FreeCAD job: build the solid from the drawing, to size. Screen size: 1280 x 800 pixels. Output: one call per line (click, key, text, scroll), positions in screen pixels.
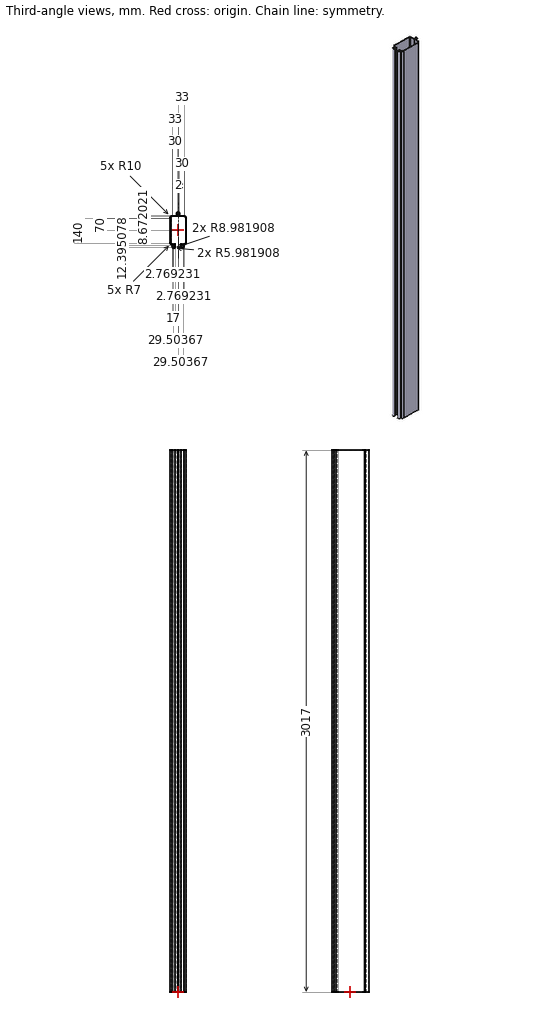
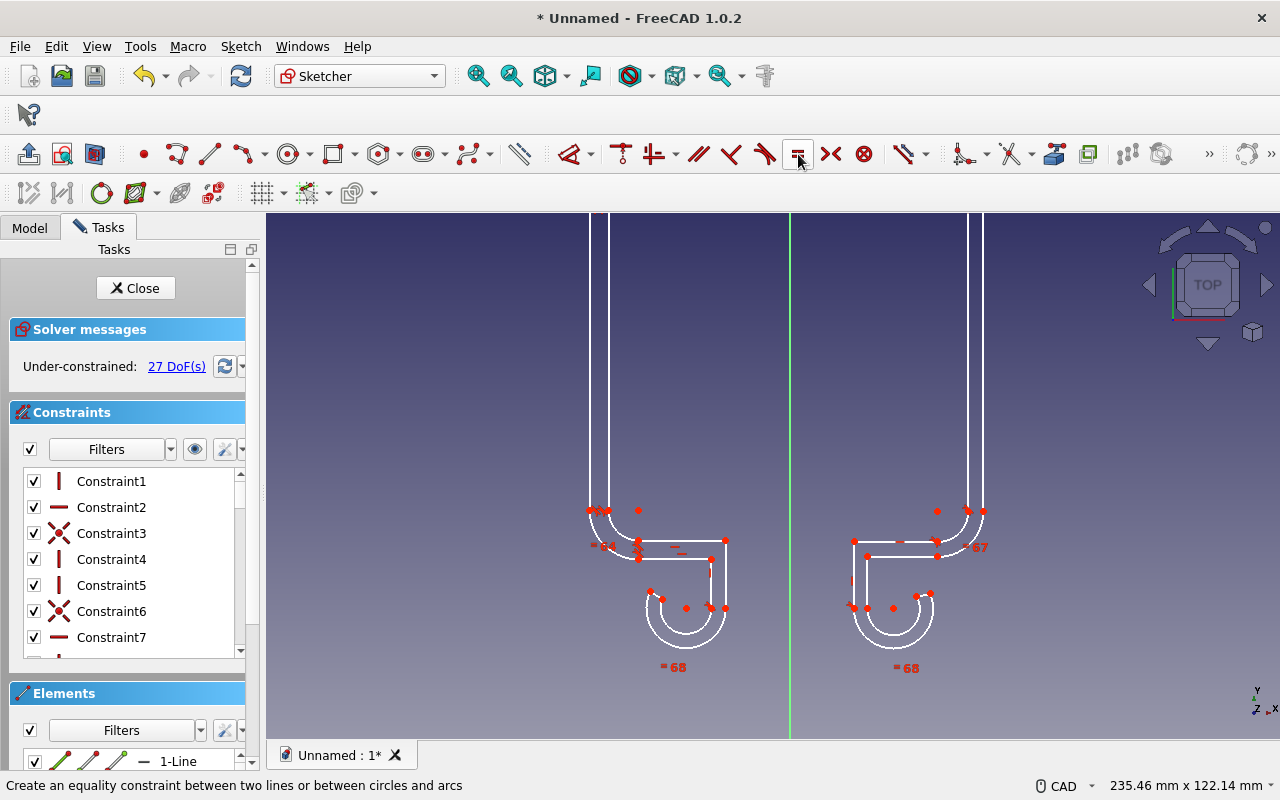
click(666, 625)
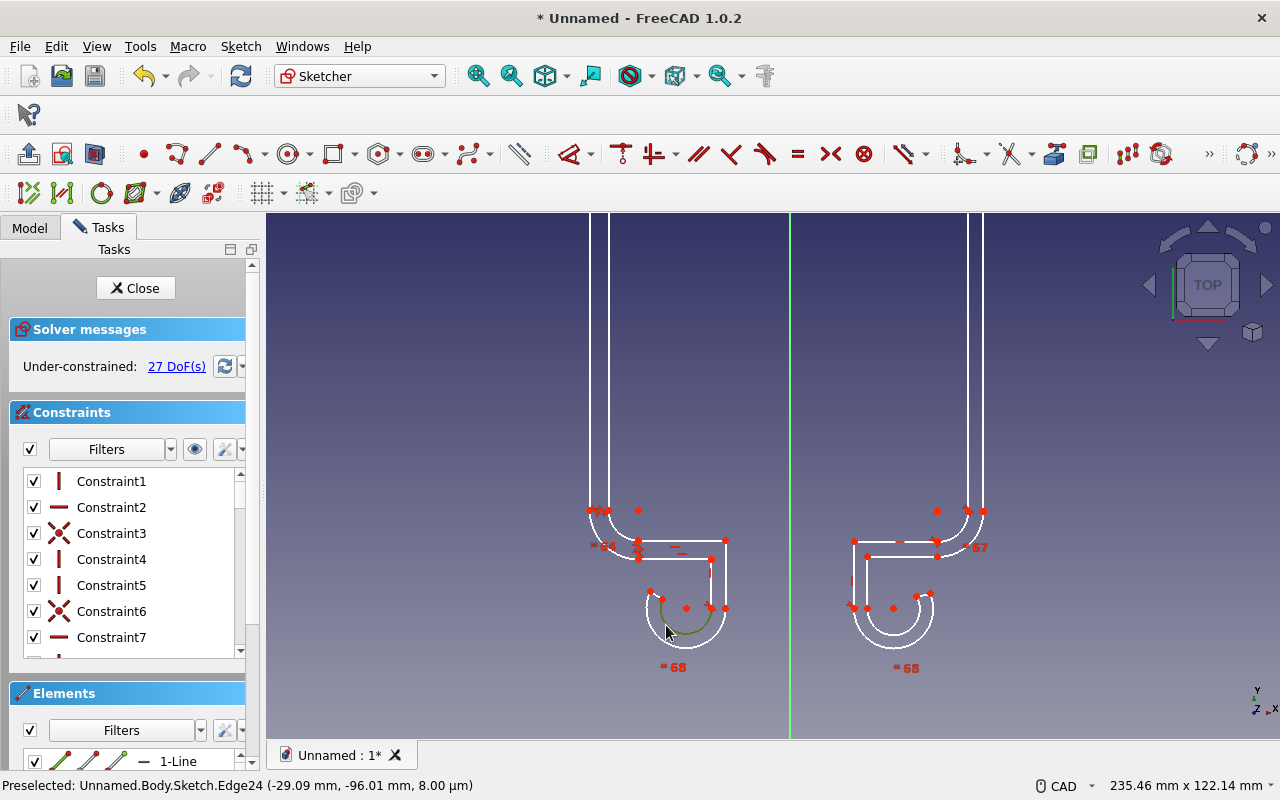
click(881, 632)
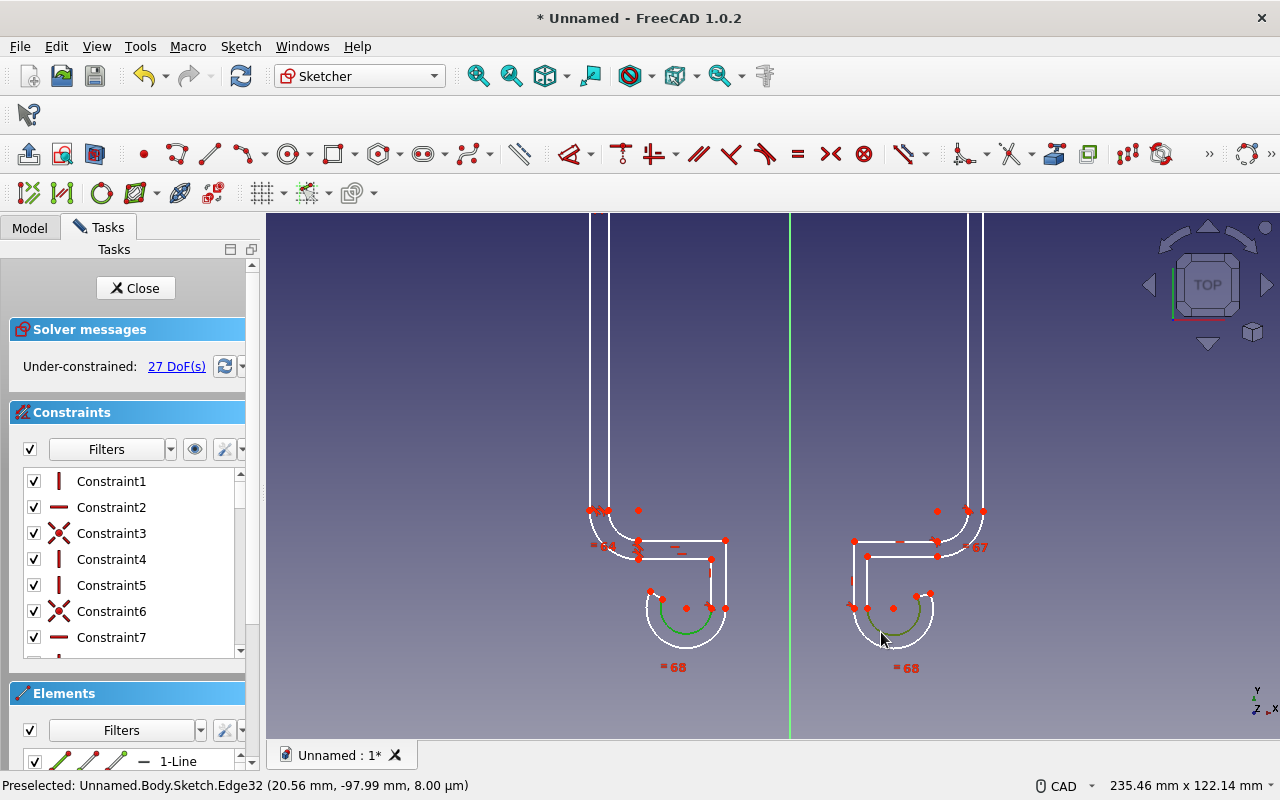
click(798, 154)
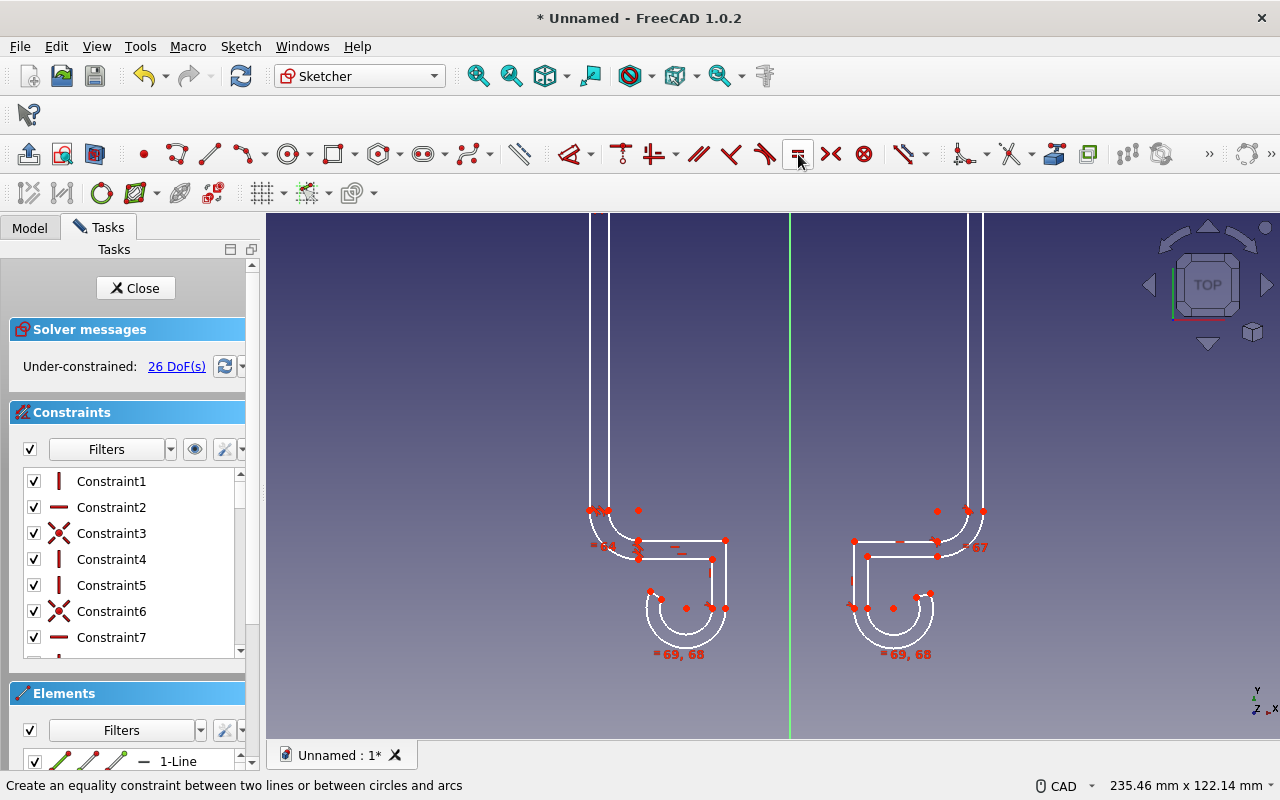
click(595, 533)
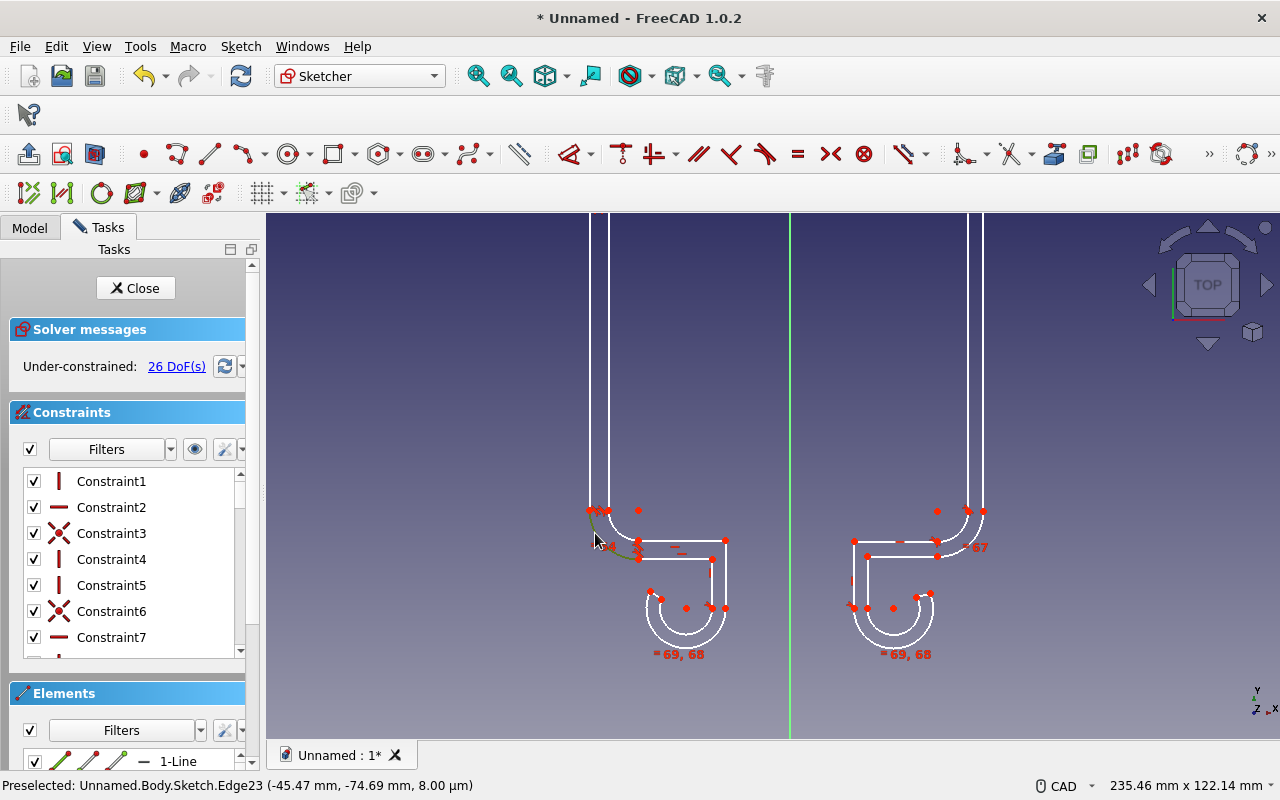
click(959, 552)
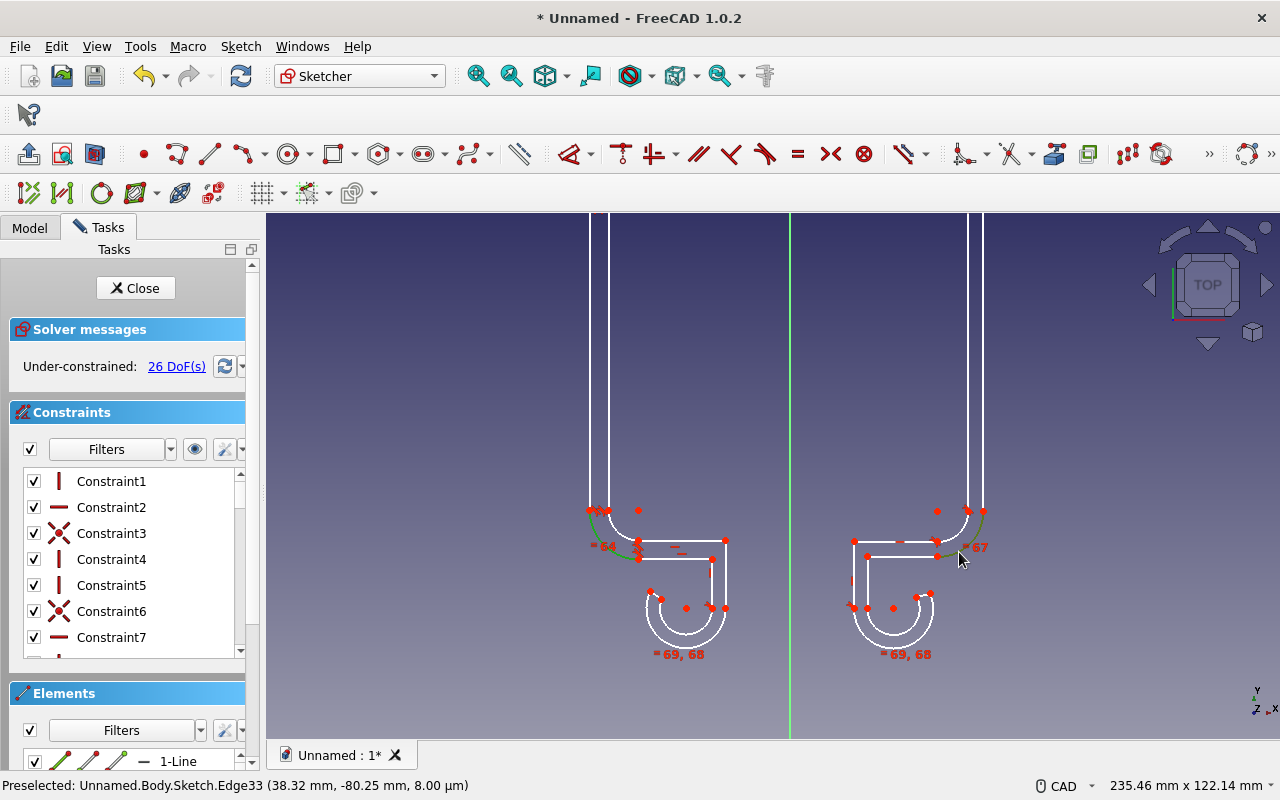
scroll(655, 633, down, 5)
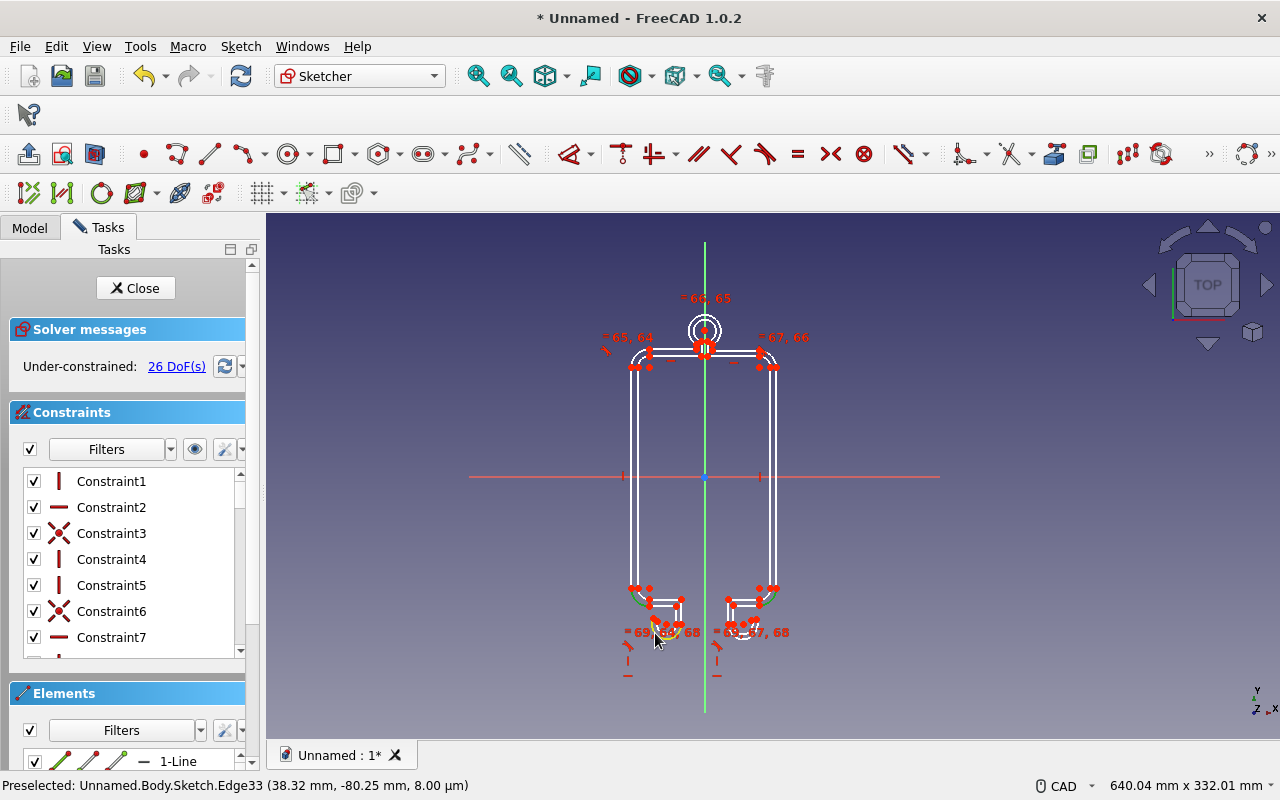
scroll(719, 323, up, 6)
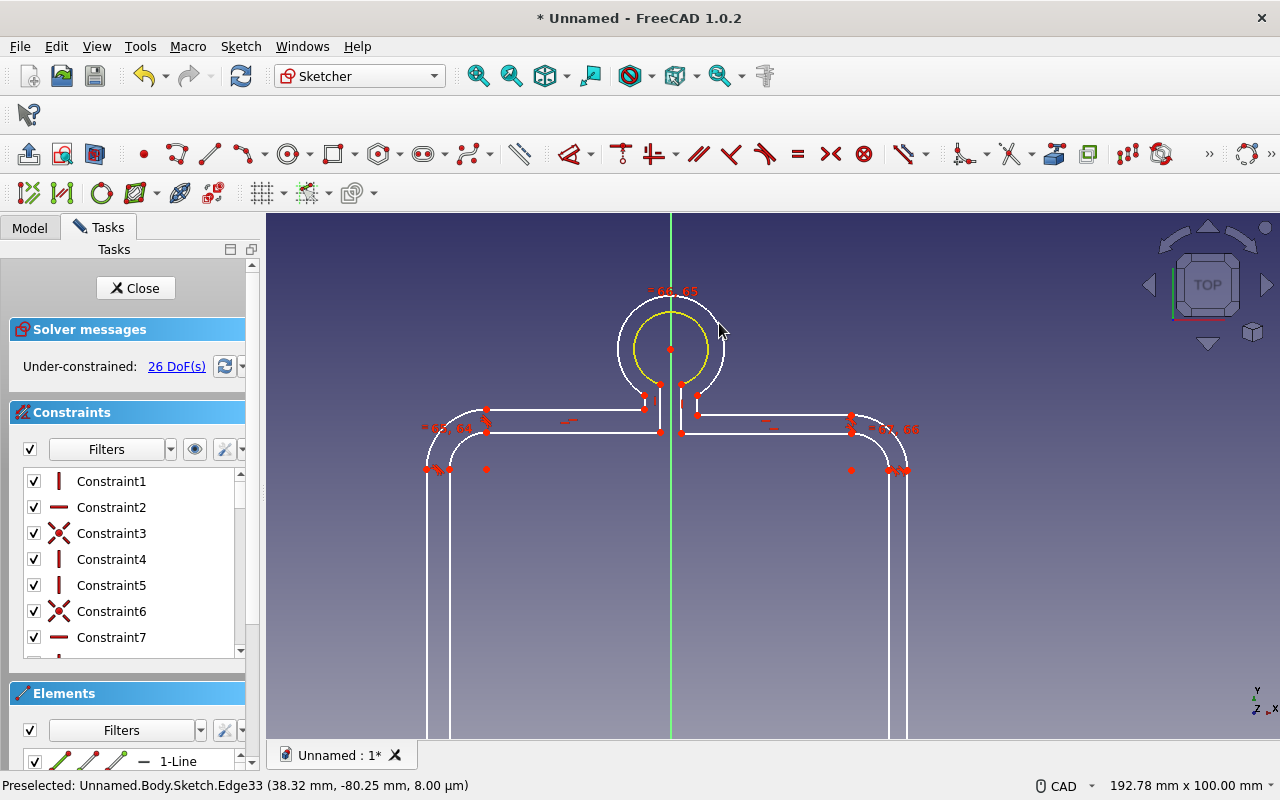
click(717, 323)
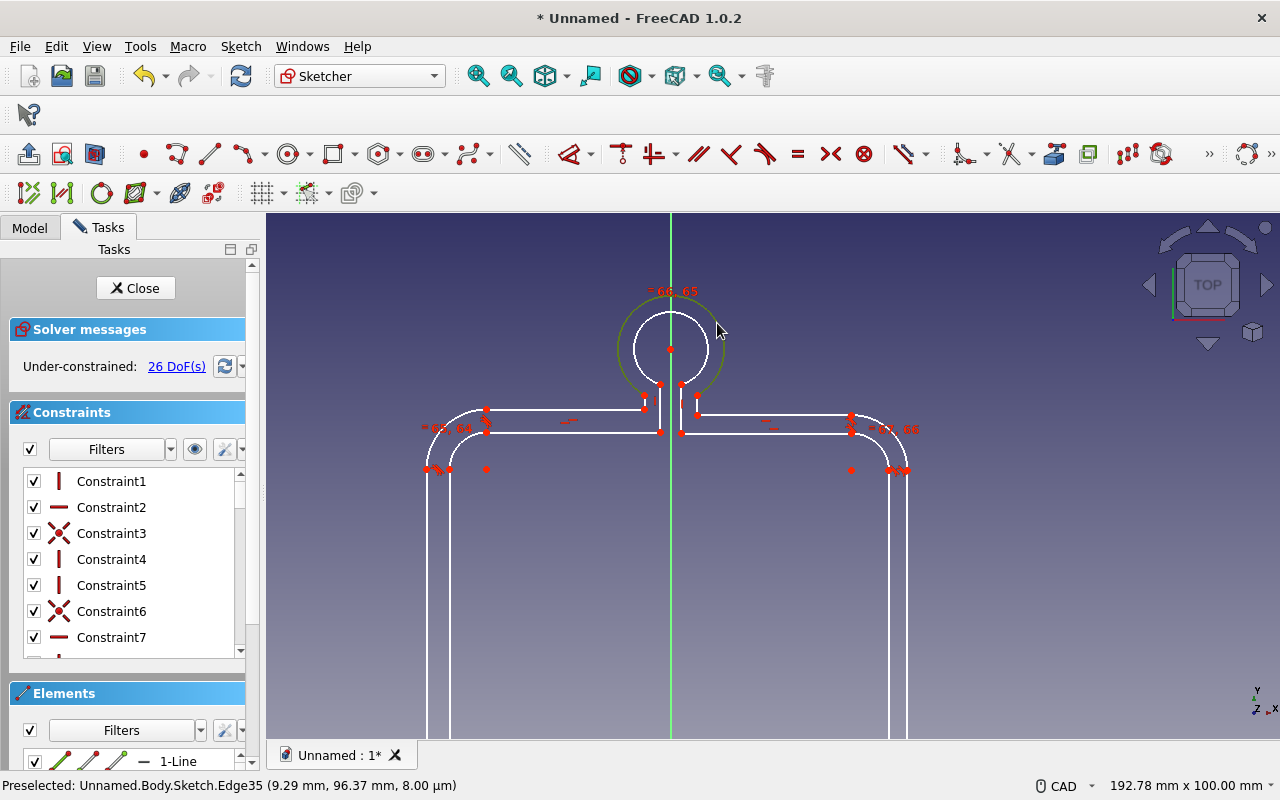
click(798, 154)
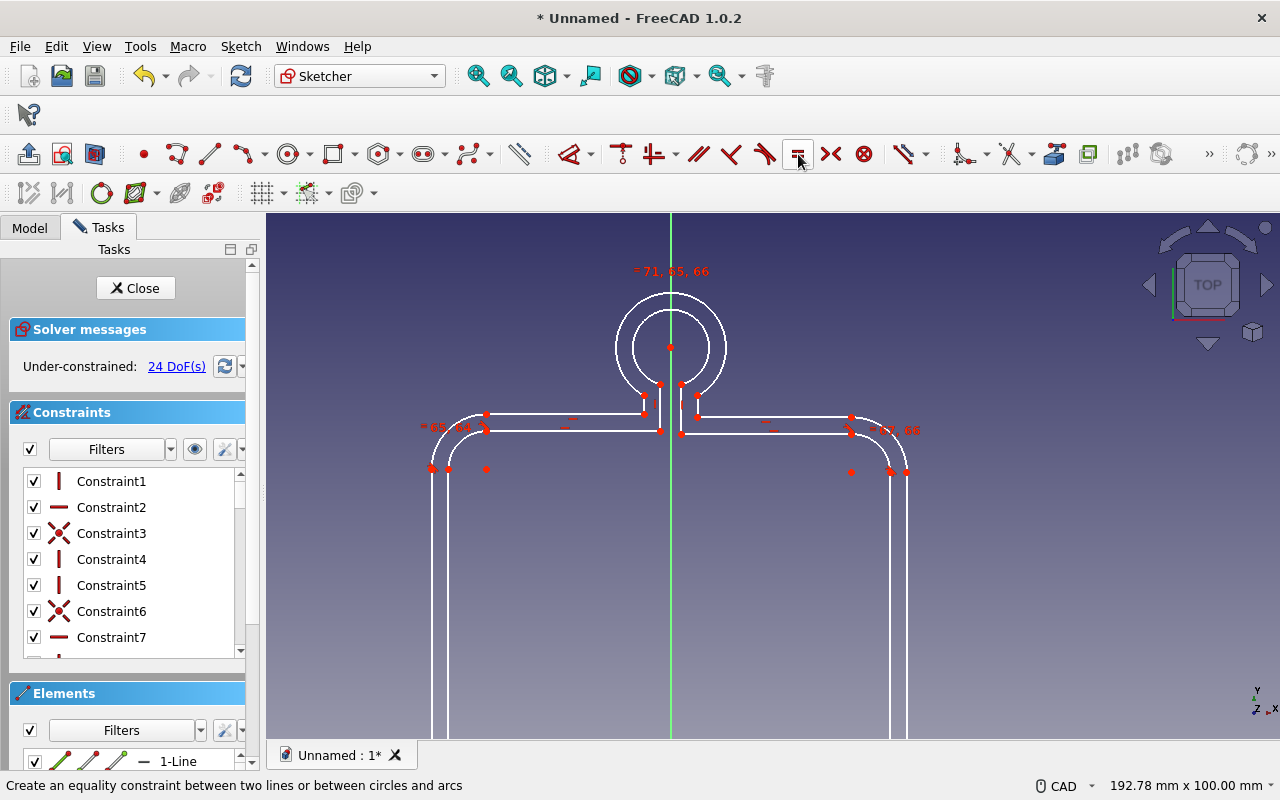
click(671, 348)